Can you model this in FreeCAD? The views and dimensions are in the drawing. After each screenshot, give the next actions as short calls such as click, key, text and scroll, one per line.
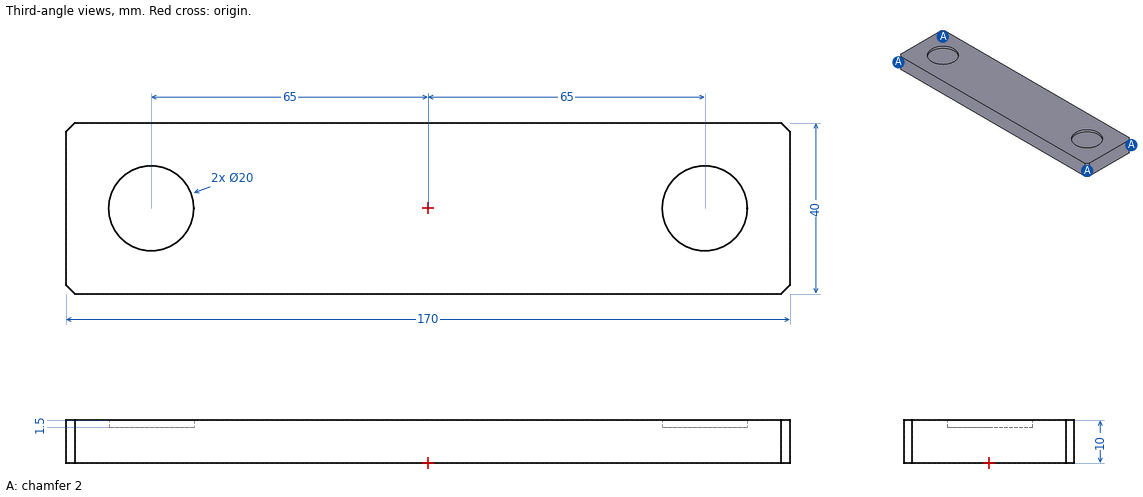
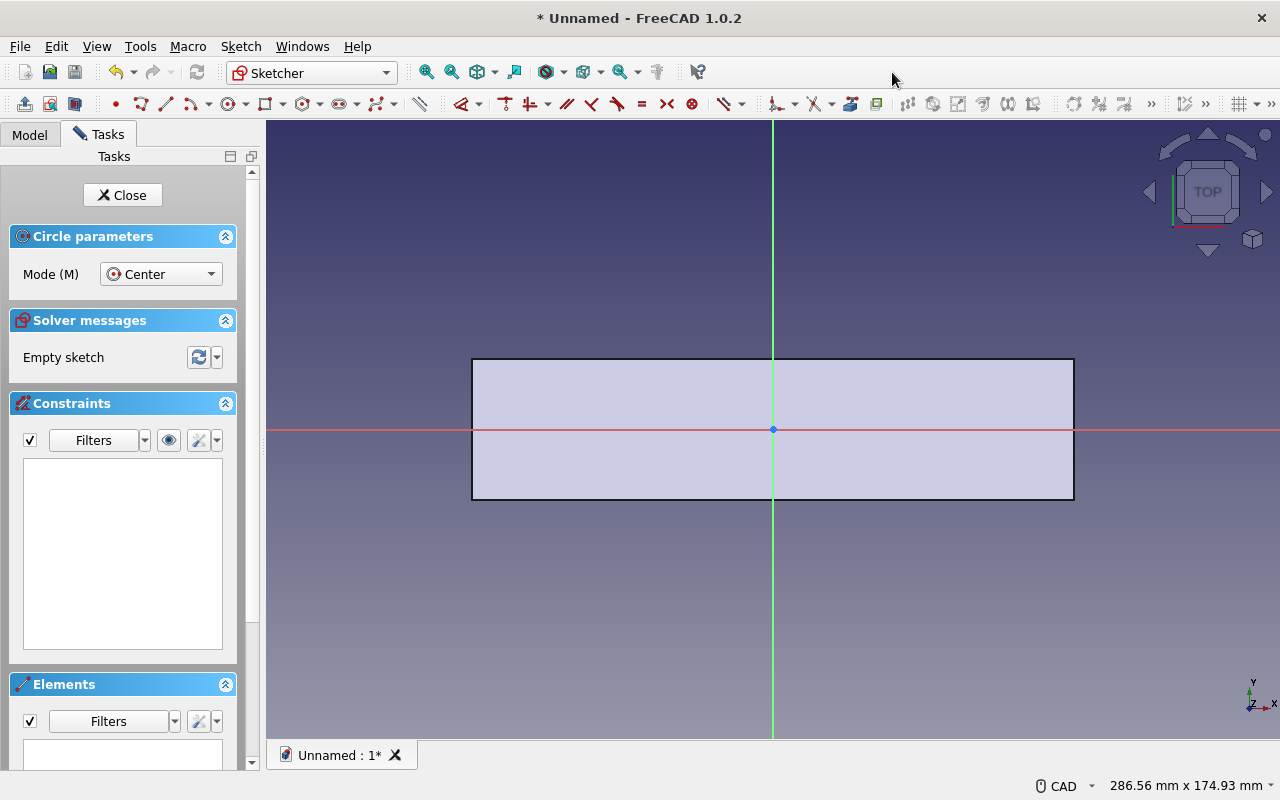
click(543, 430)
click(568, 404)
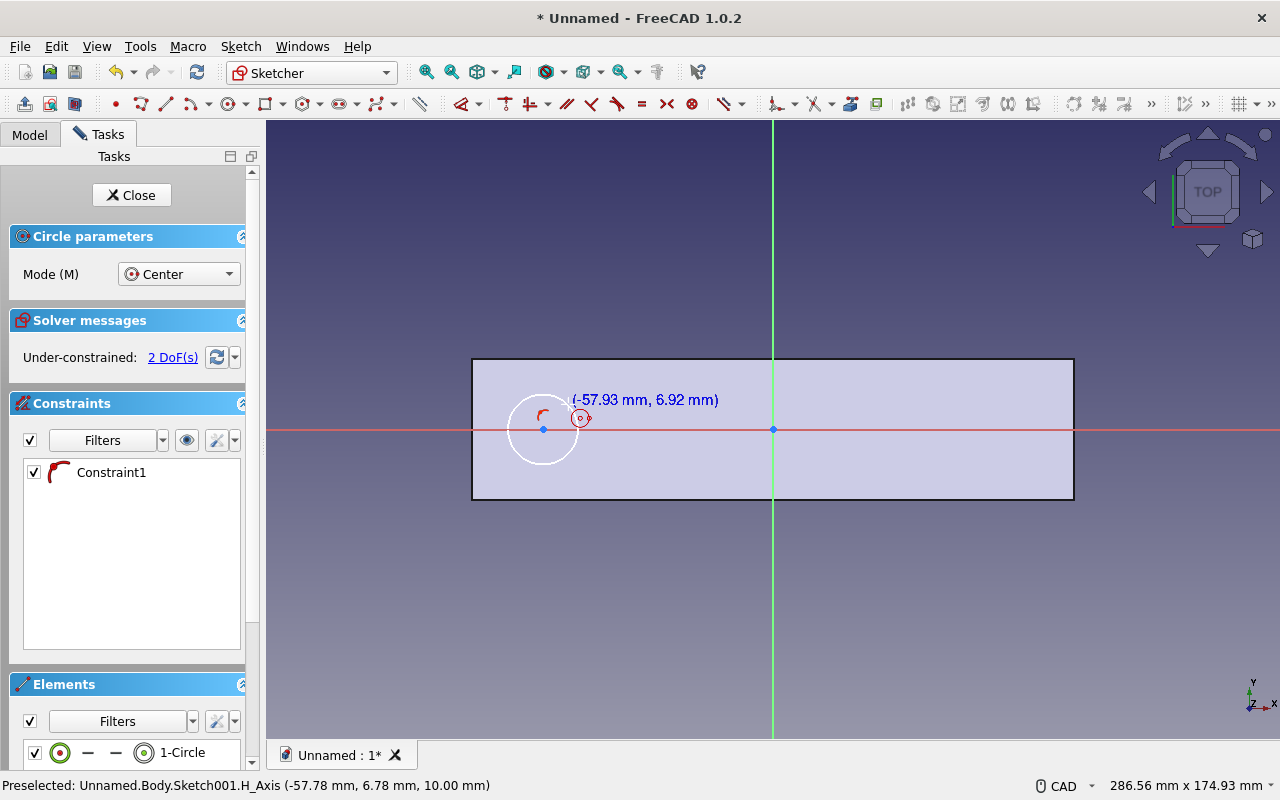
click(1003, 430)
click(1028, 404)
key(Escape)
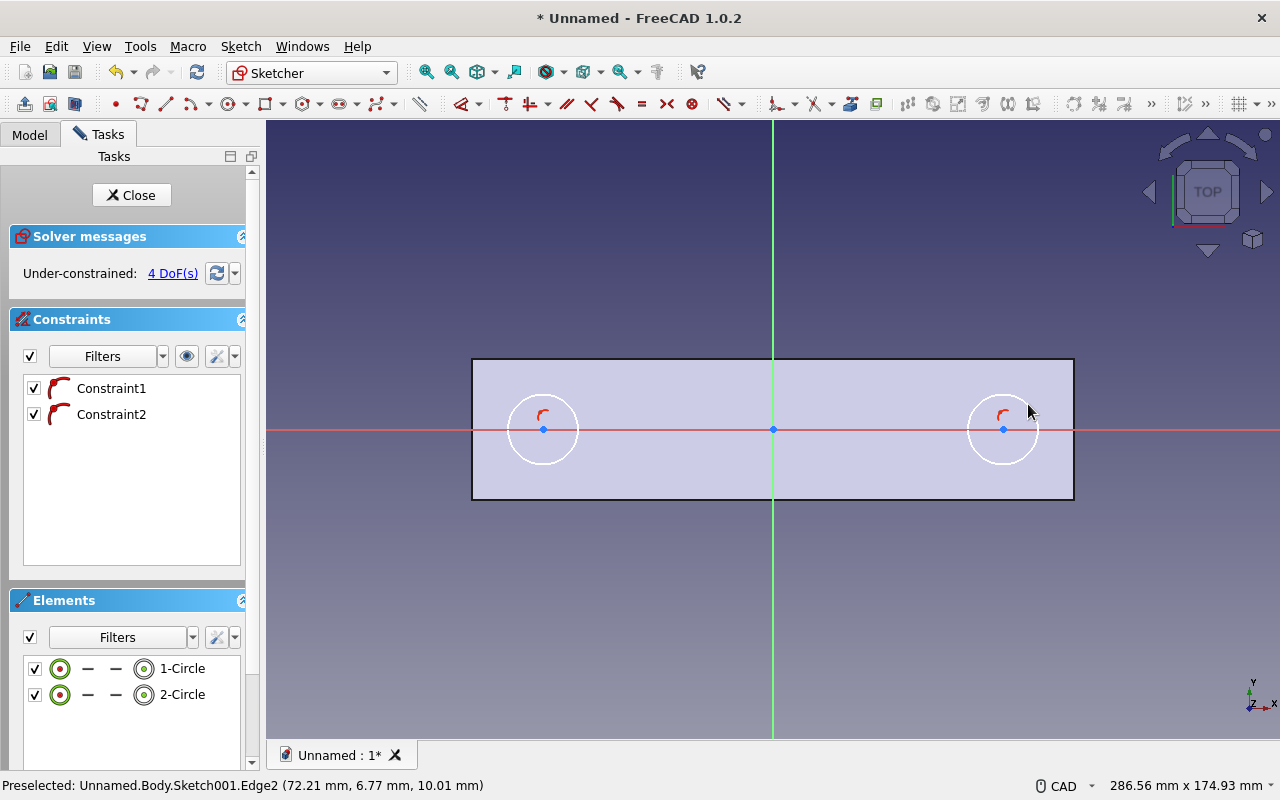
click(568, 405)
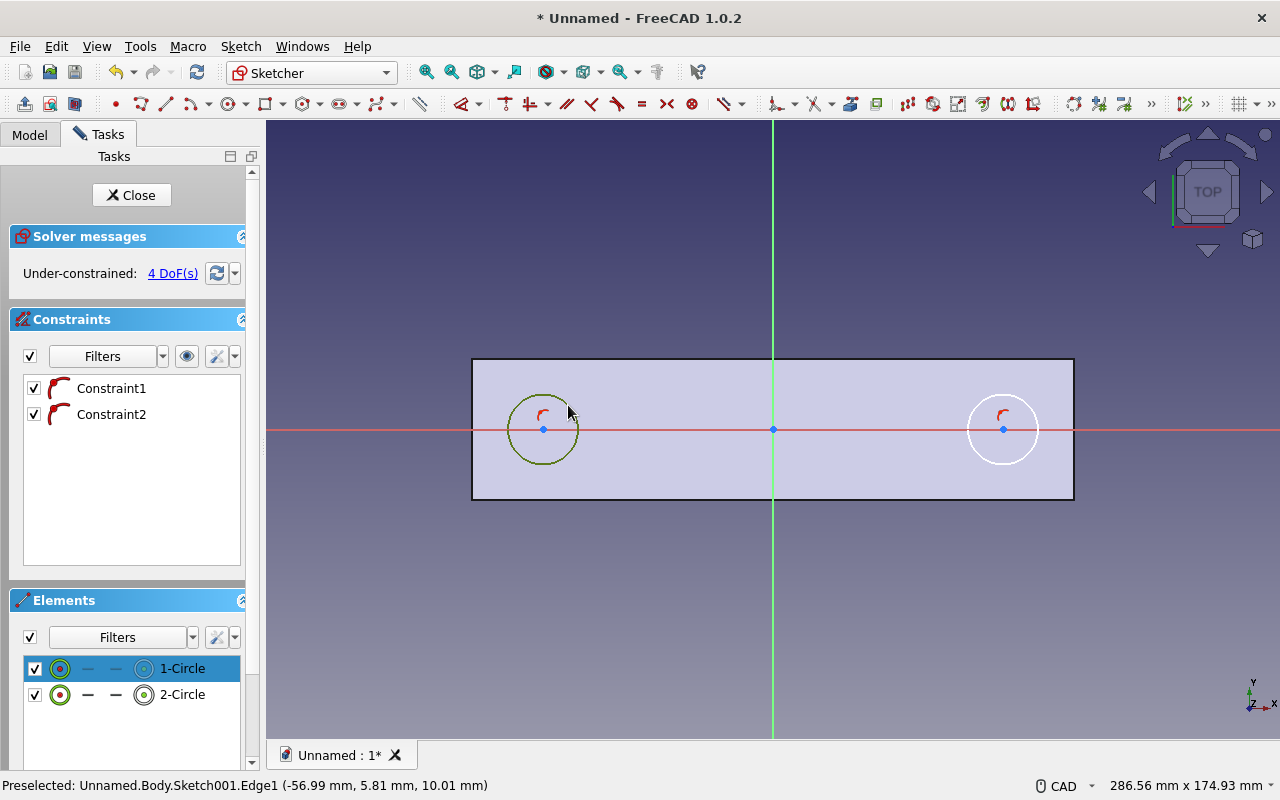
click(1028, 405)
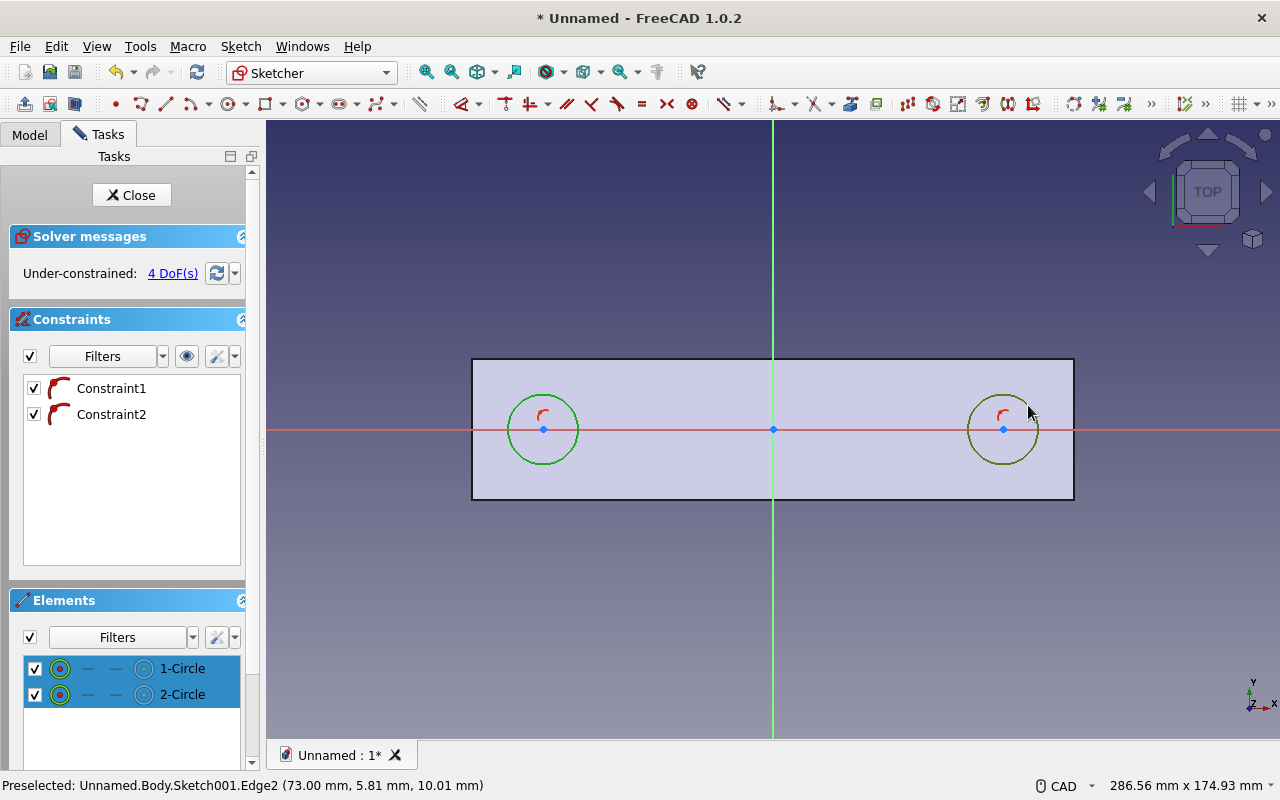
click(642, 104)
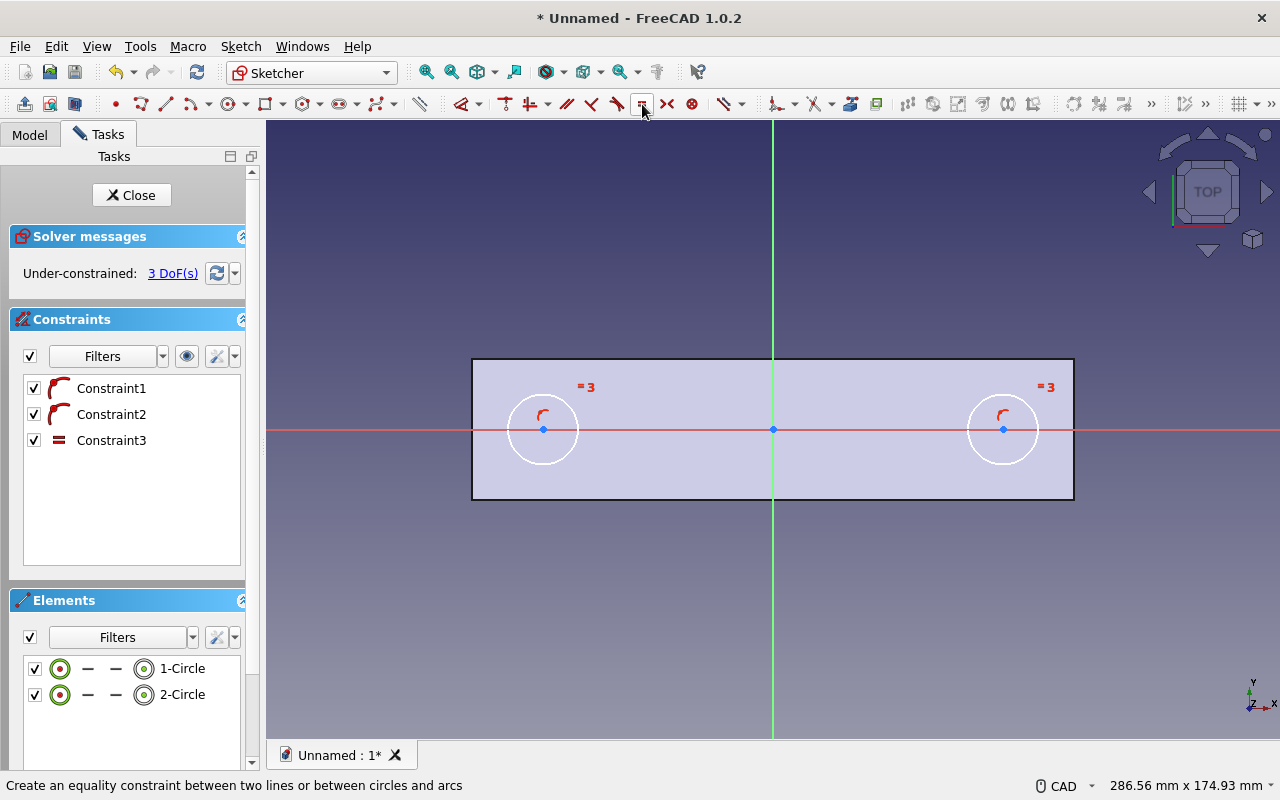
key(d)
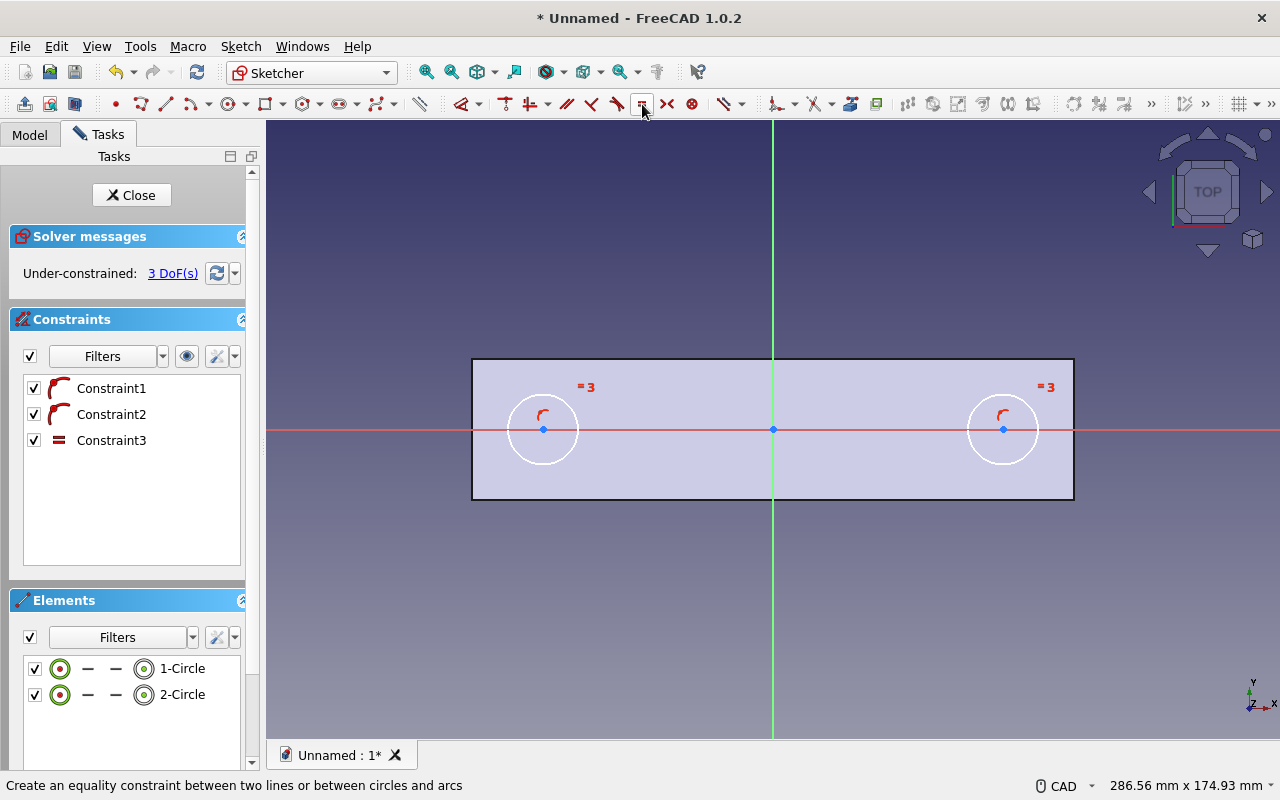
click(568, 405)
click(591, 383)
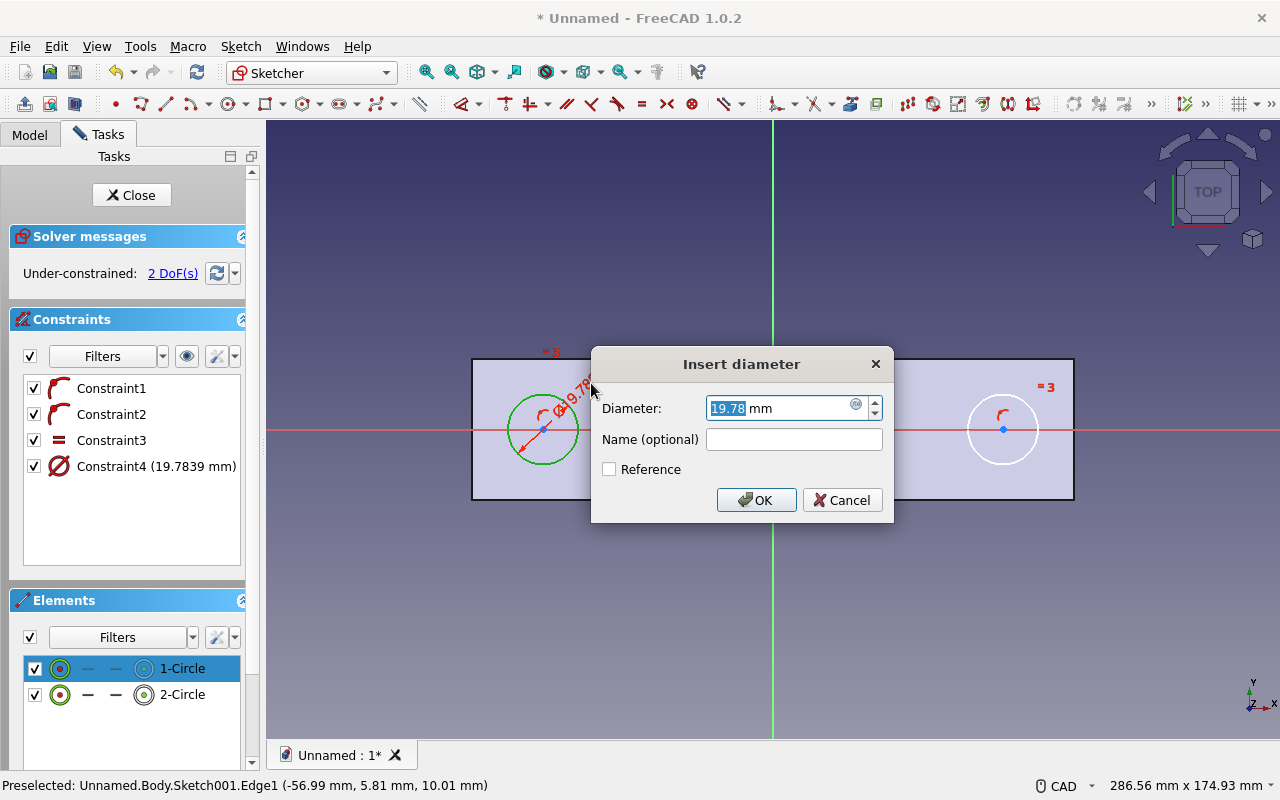
text(20)
key(Return)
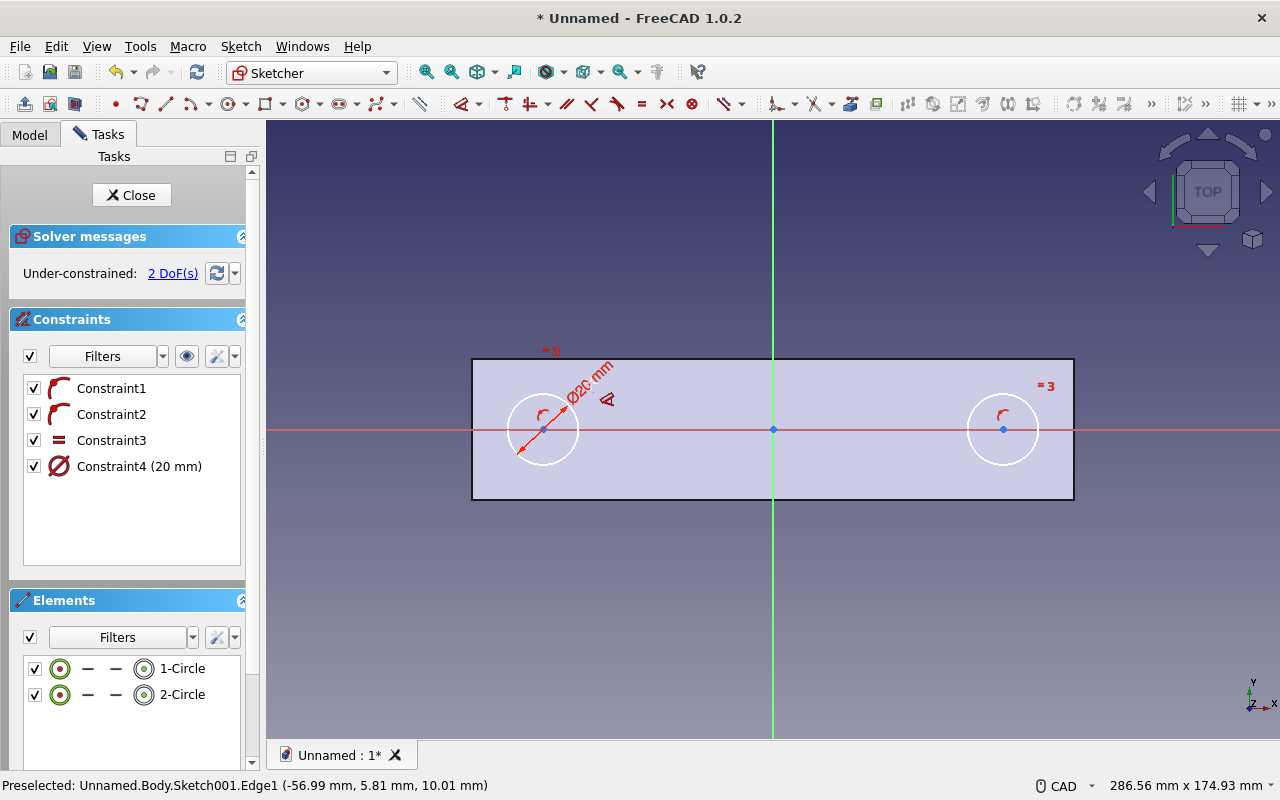
click(543, 430)
click(658, 464)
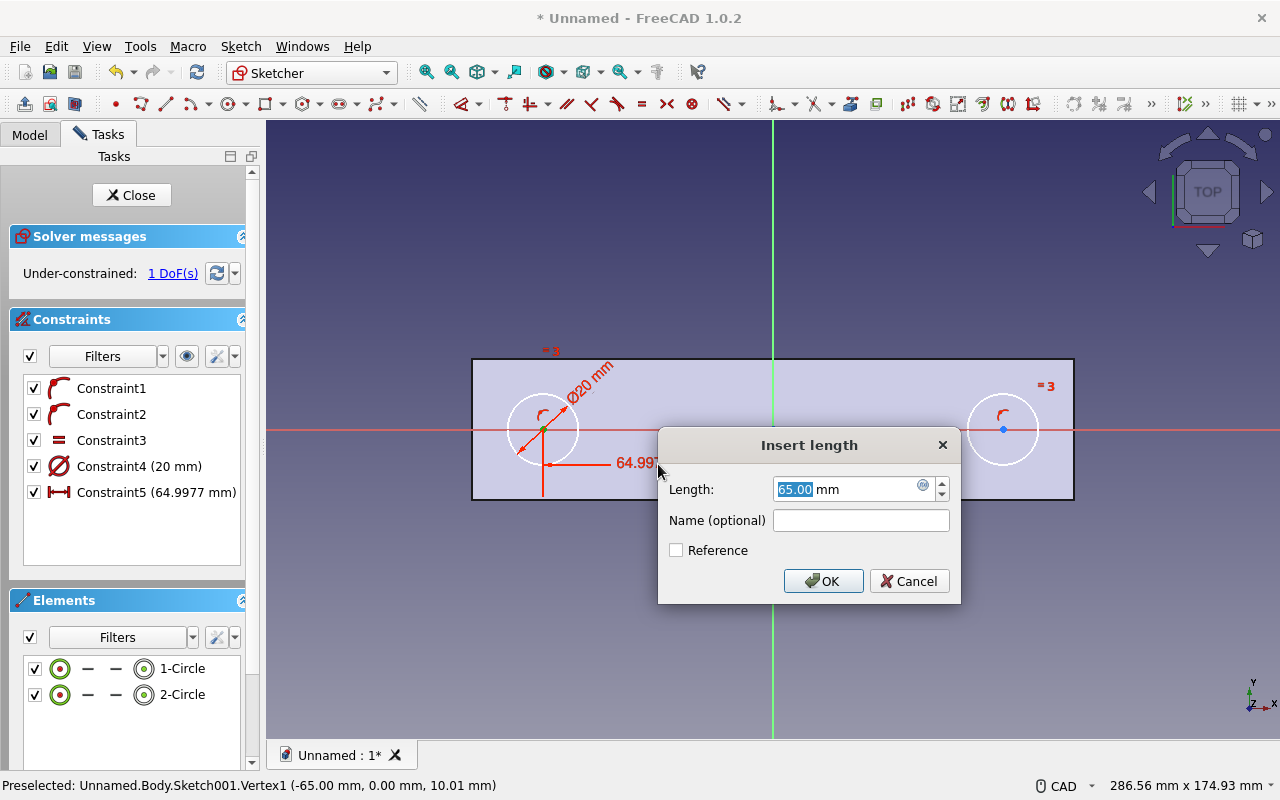
text(65)
key(Return)